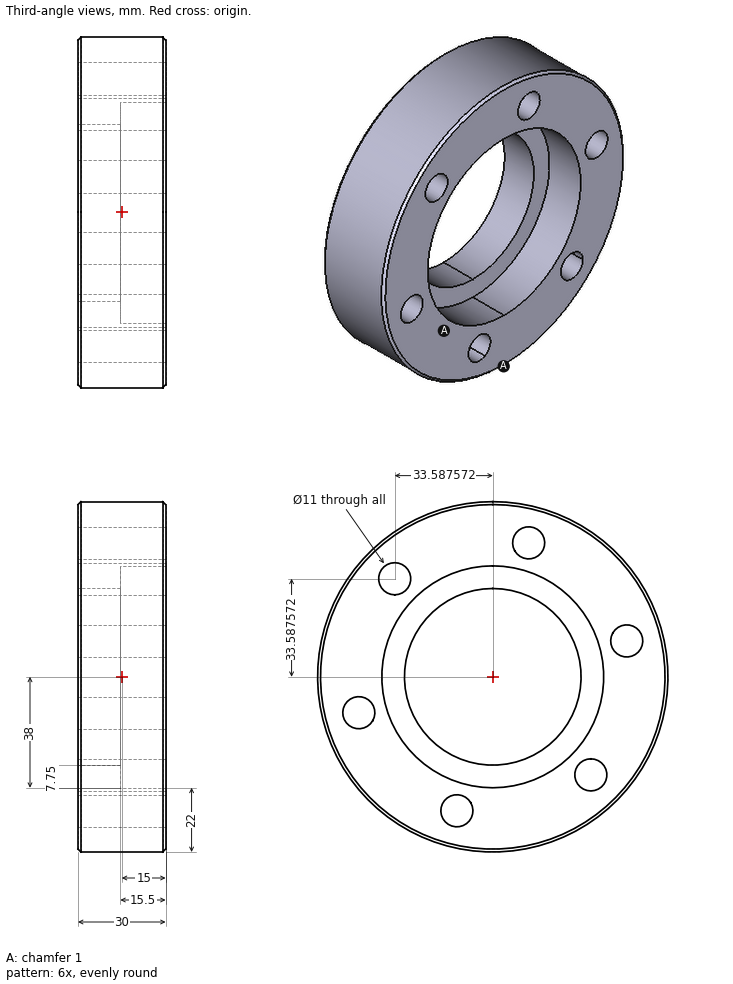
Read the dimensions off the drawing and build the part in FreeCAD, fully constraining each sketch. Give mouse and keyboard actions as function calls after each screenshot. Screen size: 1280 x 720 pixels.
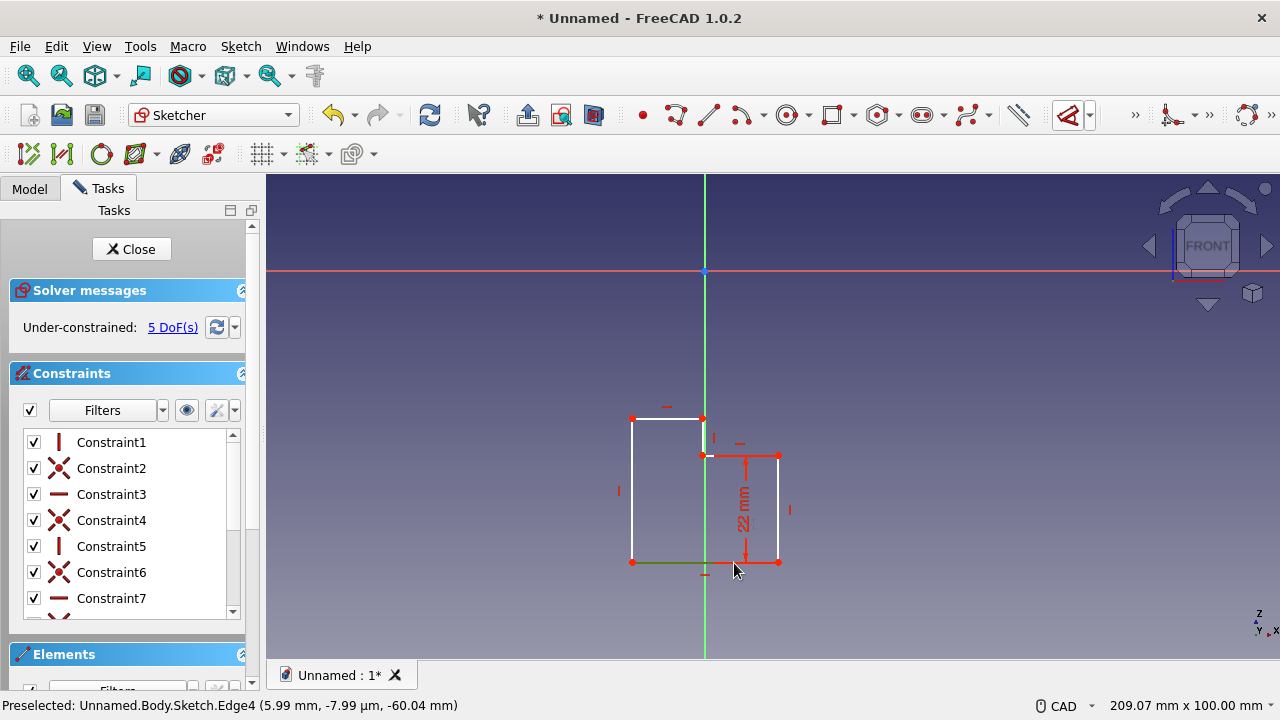
key(l)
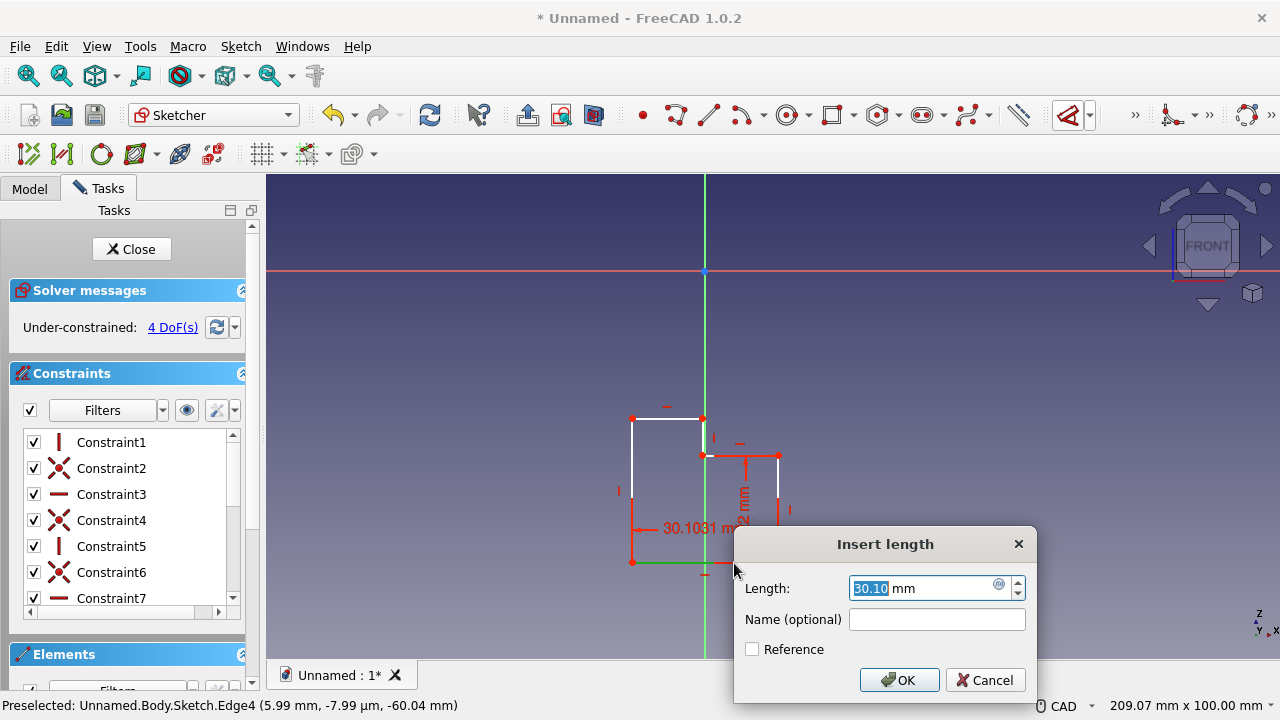
text(30)
key(Return)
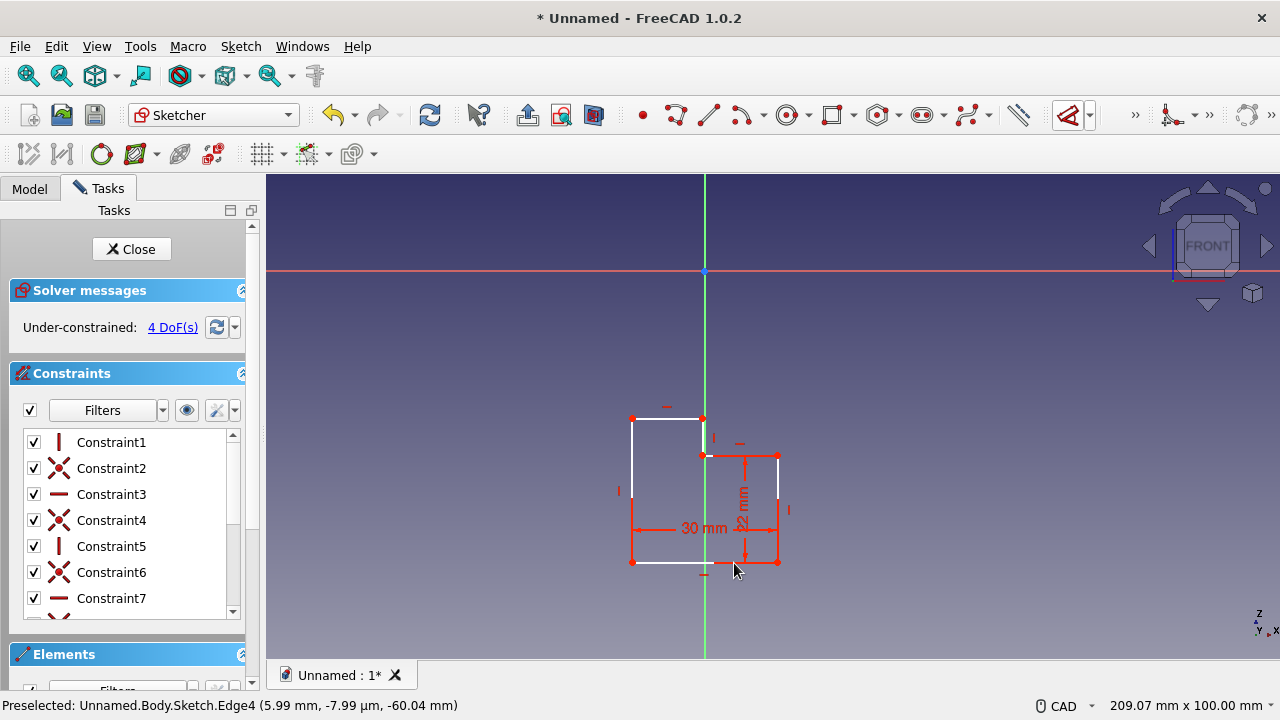
click(703, 456)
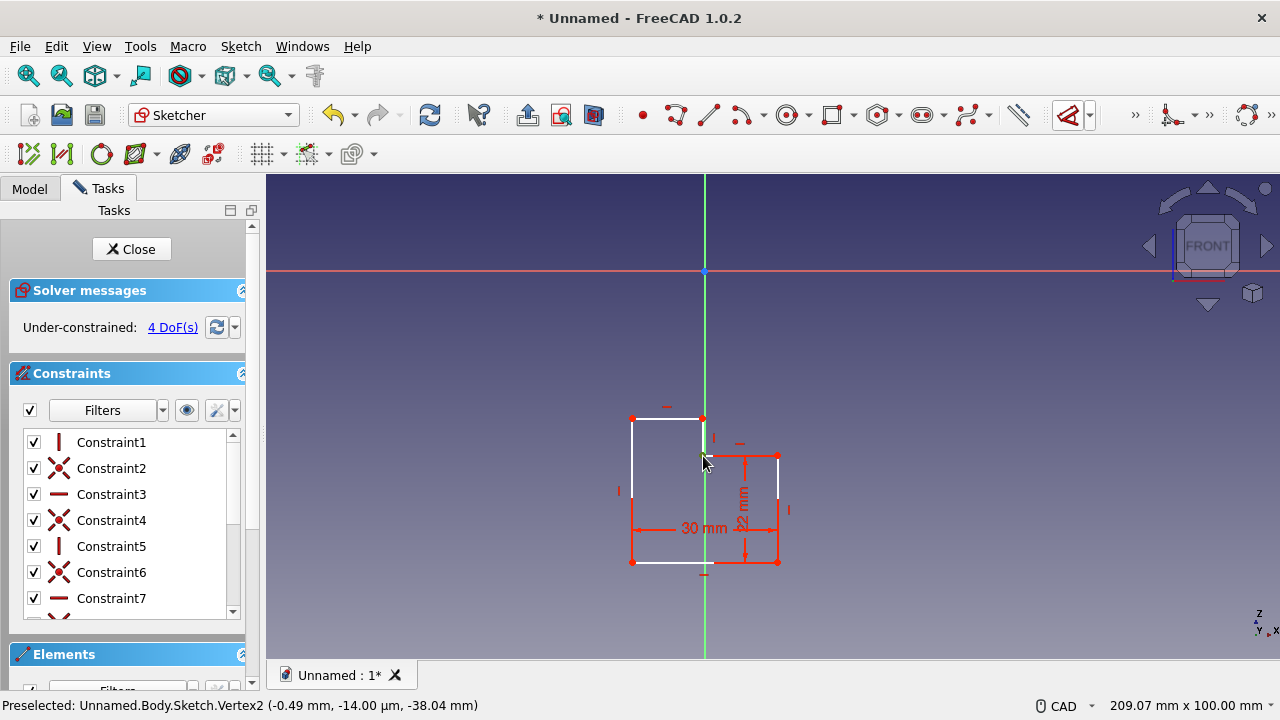
key(i)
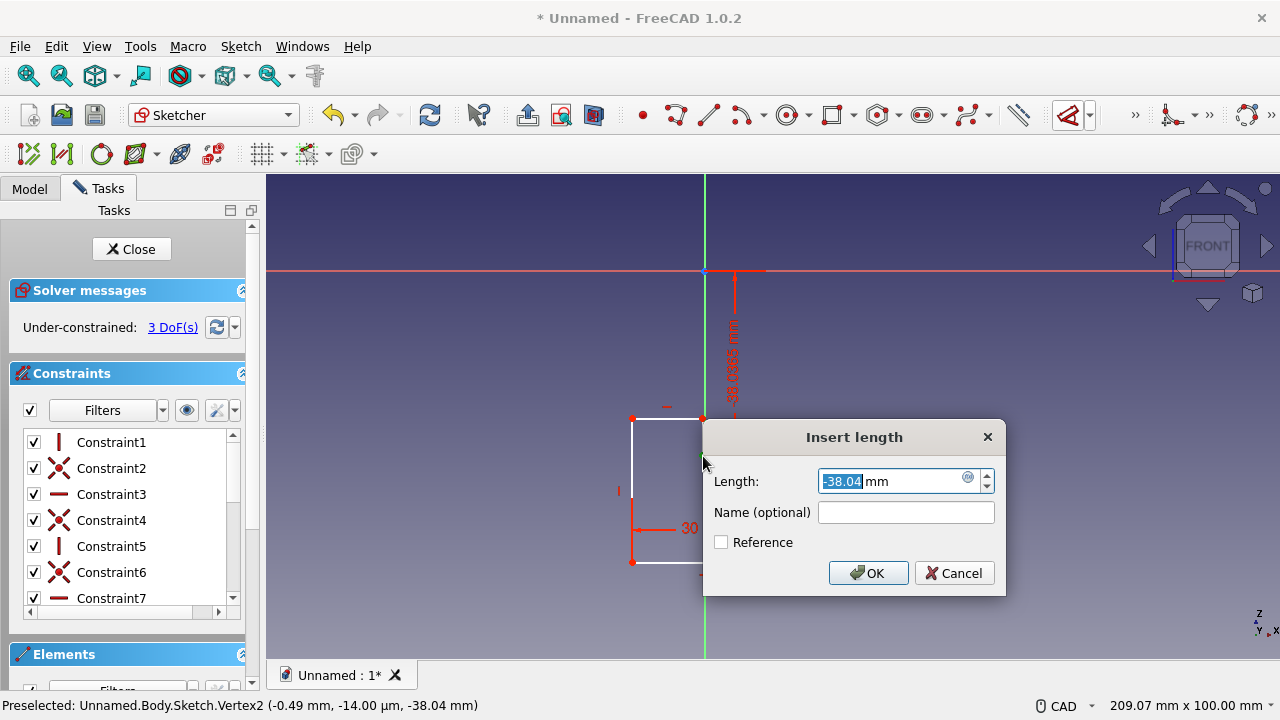
text(-38)
key(Return)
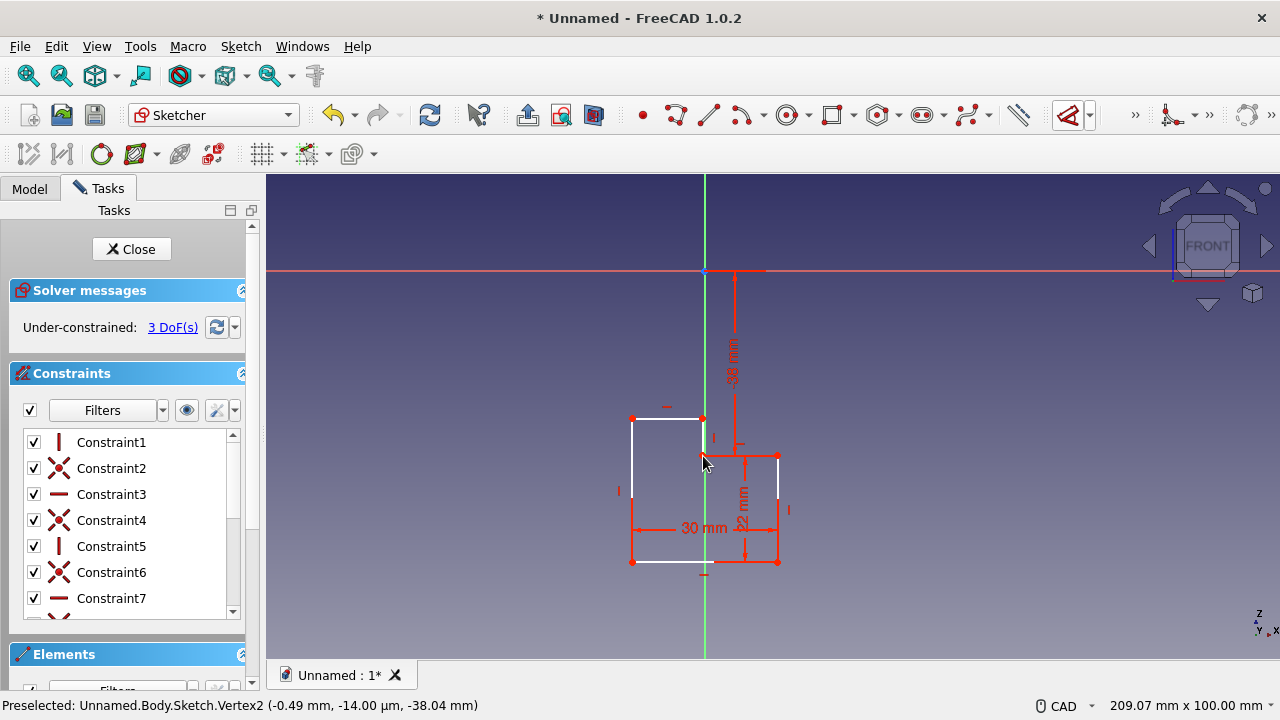
click(778, 456)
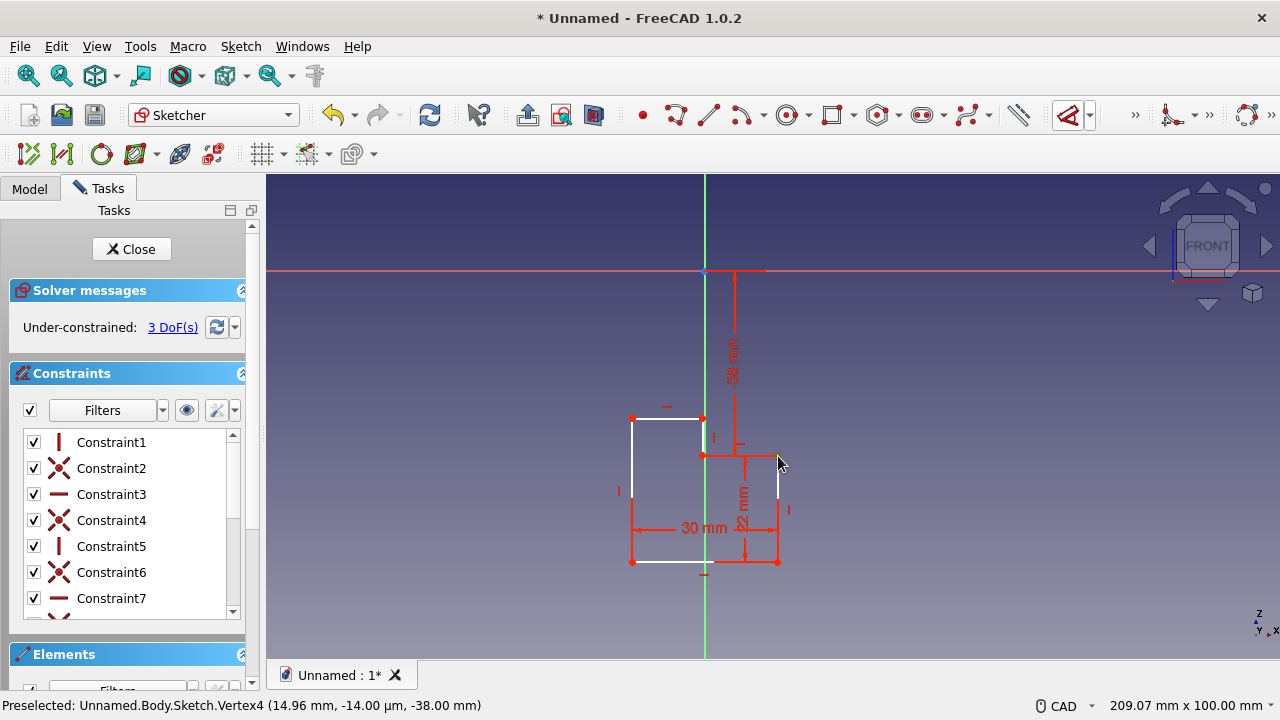
key(l)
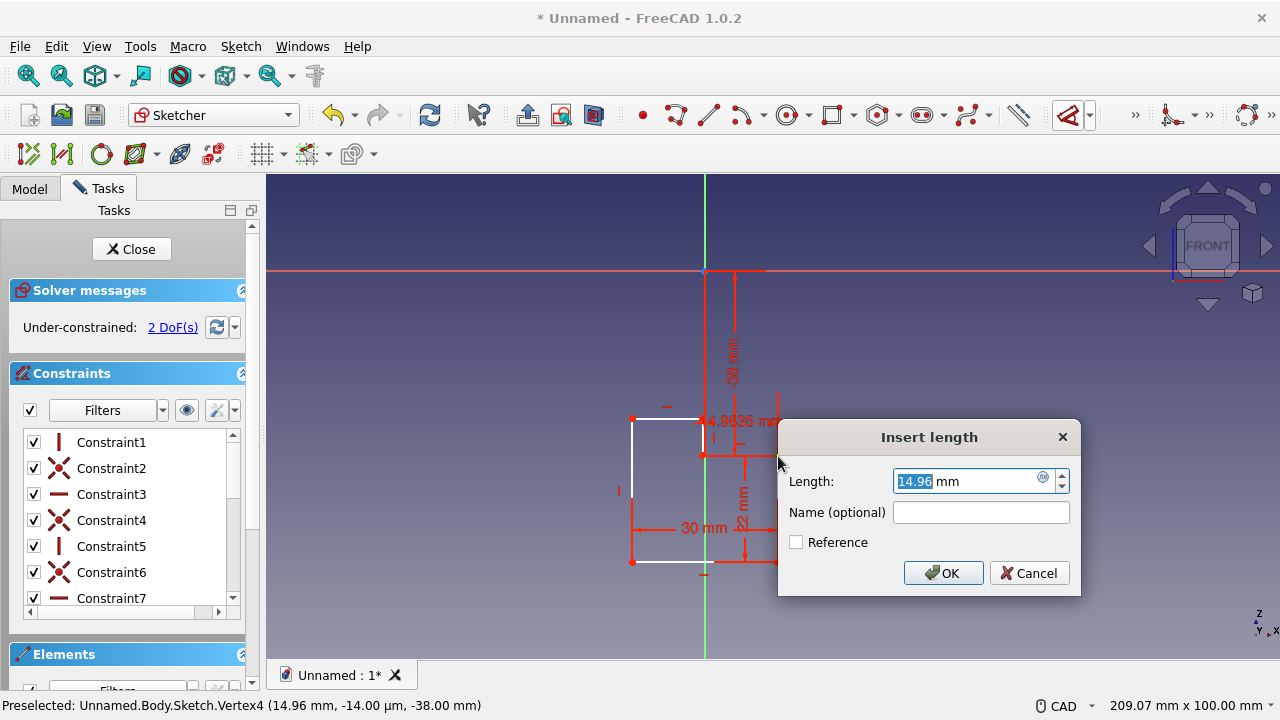
text(15)
key(Return)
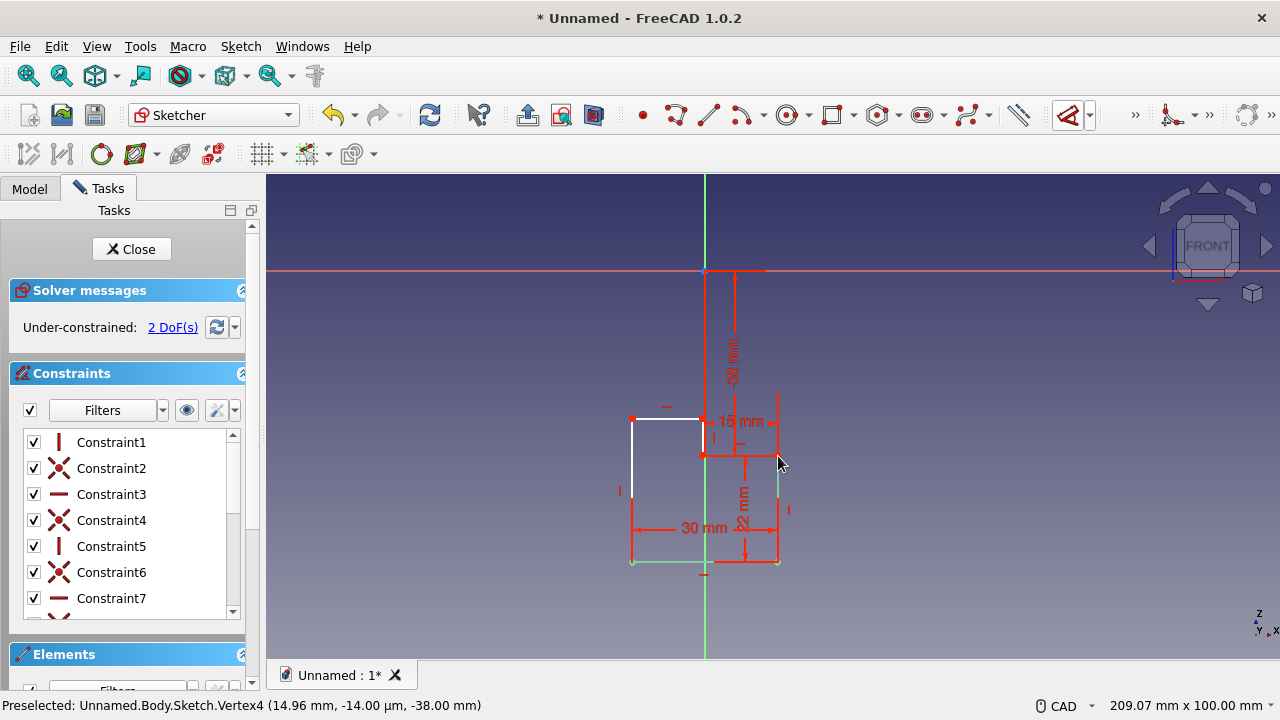
scroll(703, 430, up, 2)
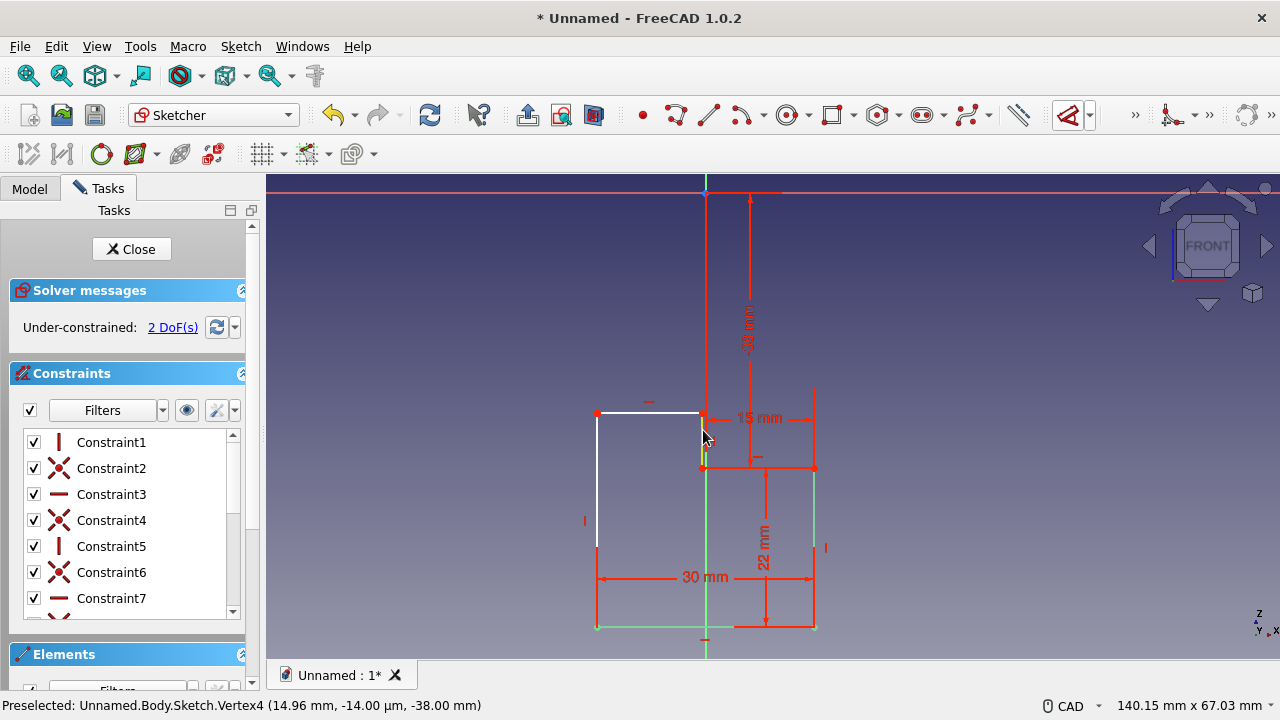
click(702, 430)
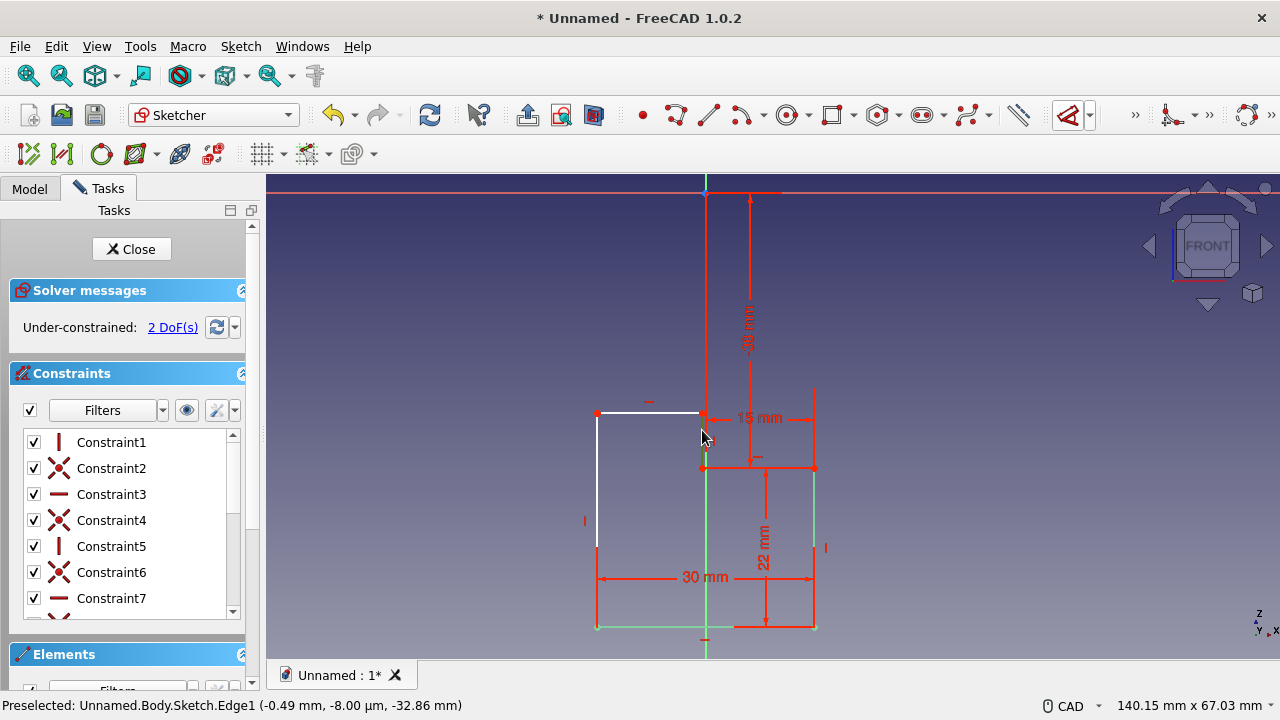
key(i)